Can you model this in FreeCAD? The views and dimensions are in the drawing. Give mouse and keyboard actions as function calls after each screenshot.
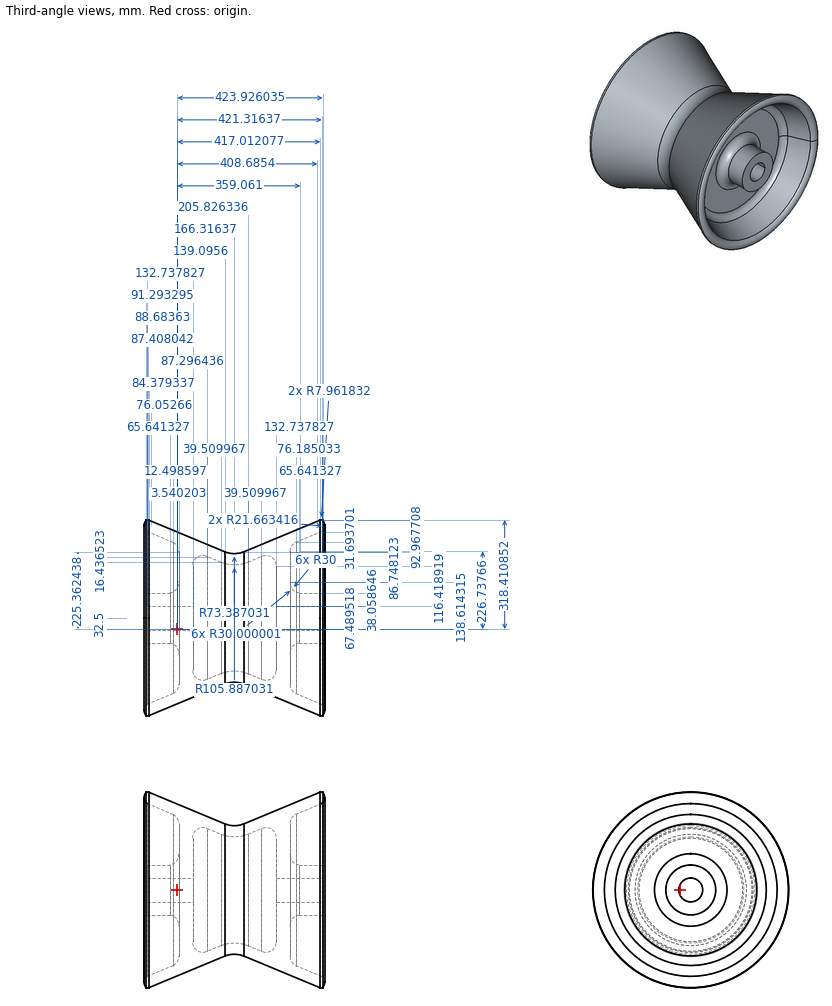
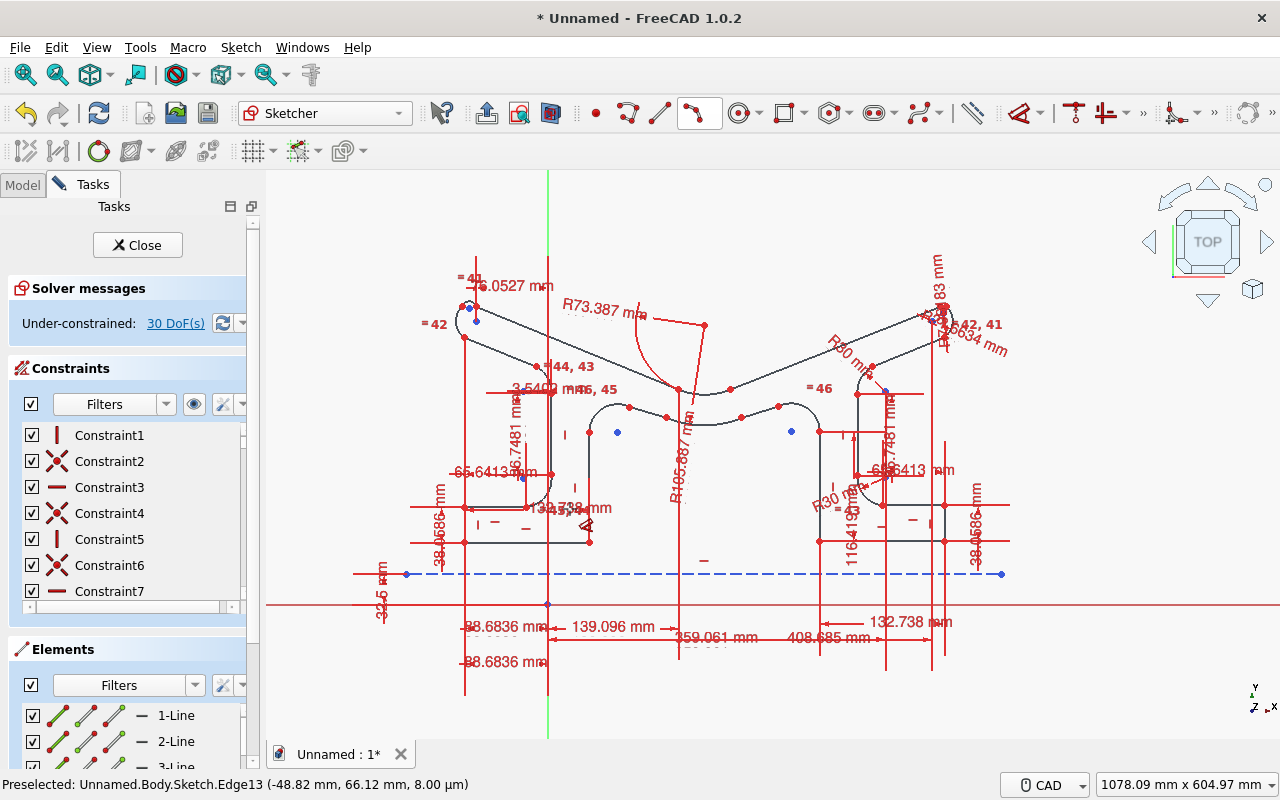
click(589, 510)
click(623, 488)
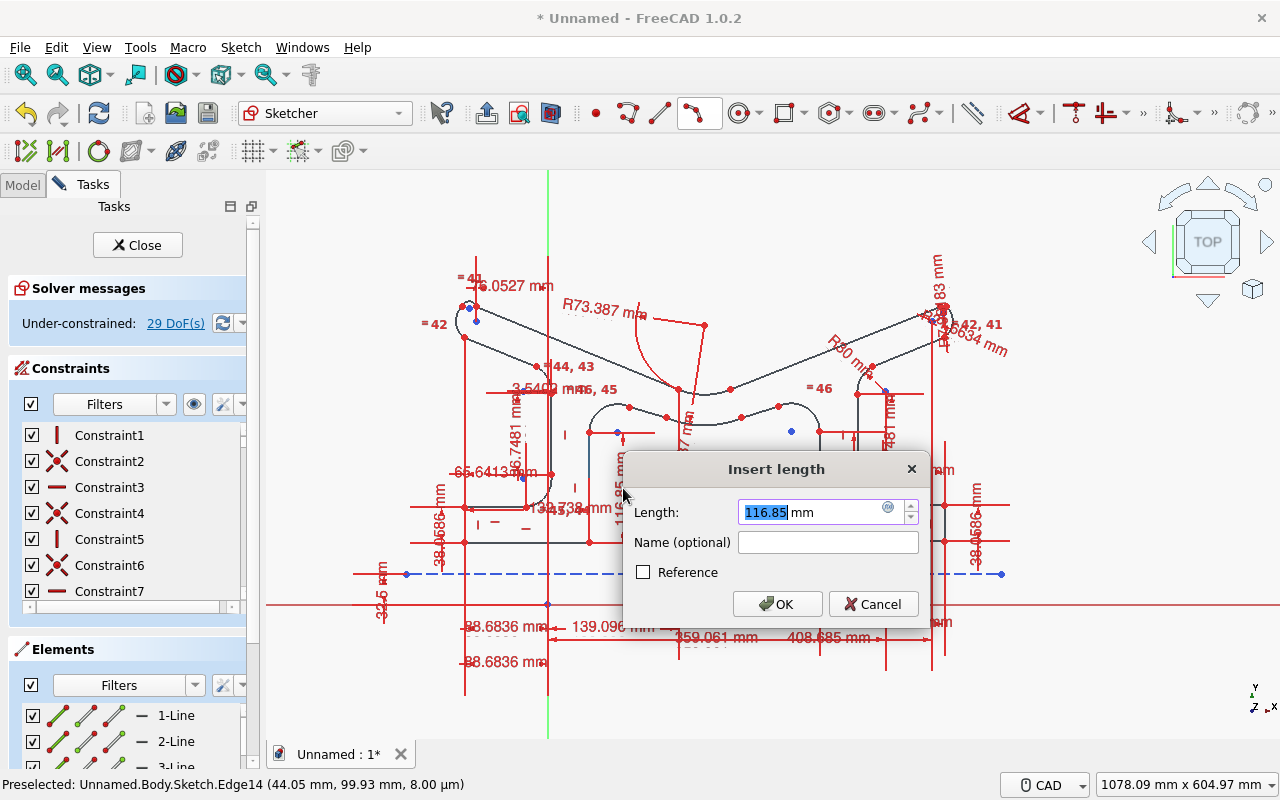
text(116.418919)
key(Return)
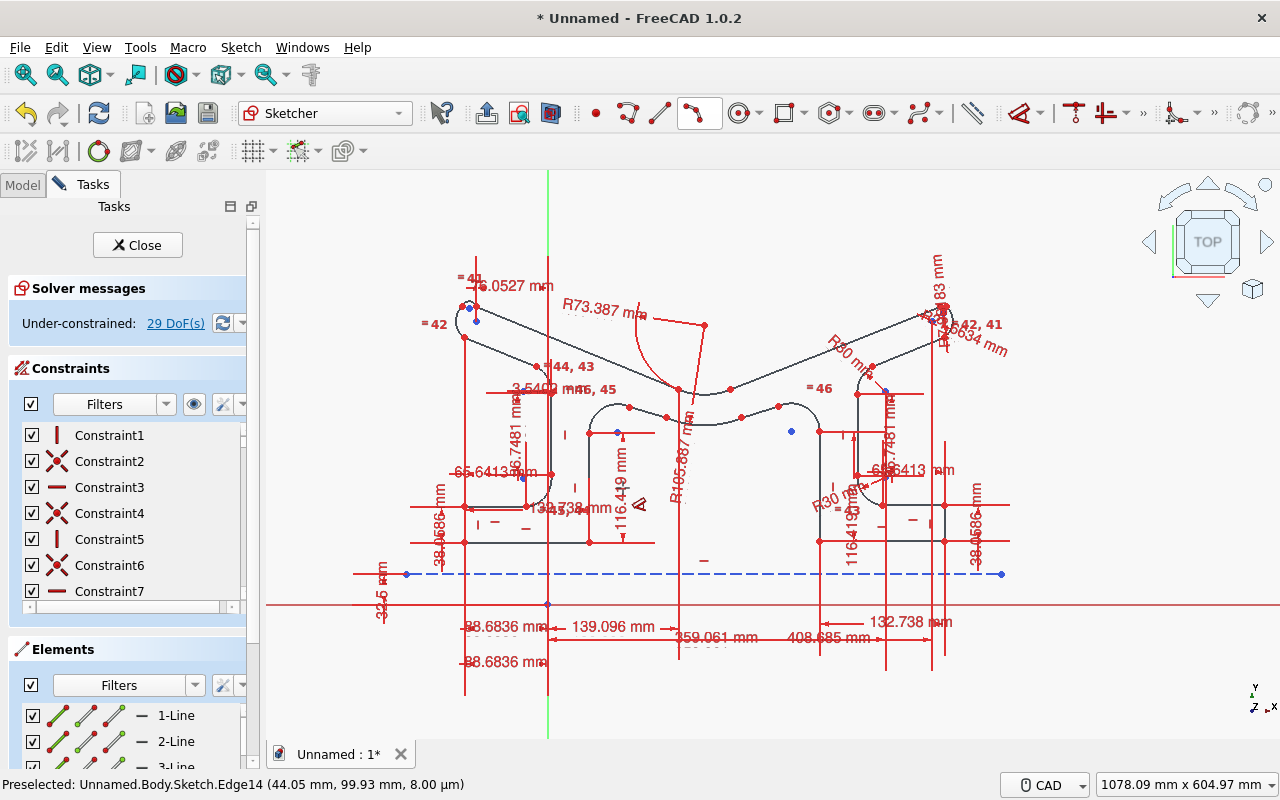
click(820, 541)
click(514, 558)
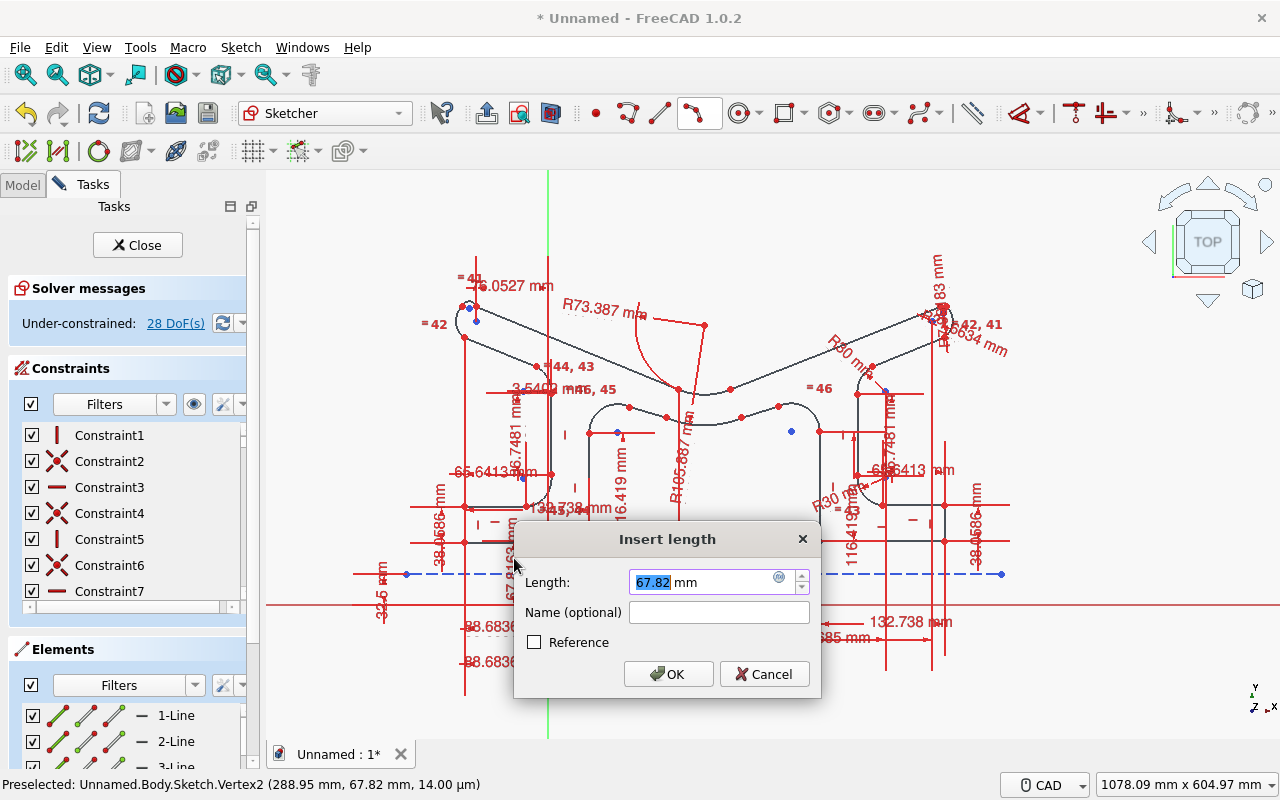
text(67.489518)
key(Return)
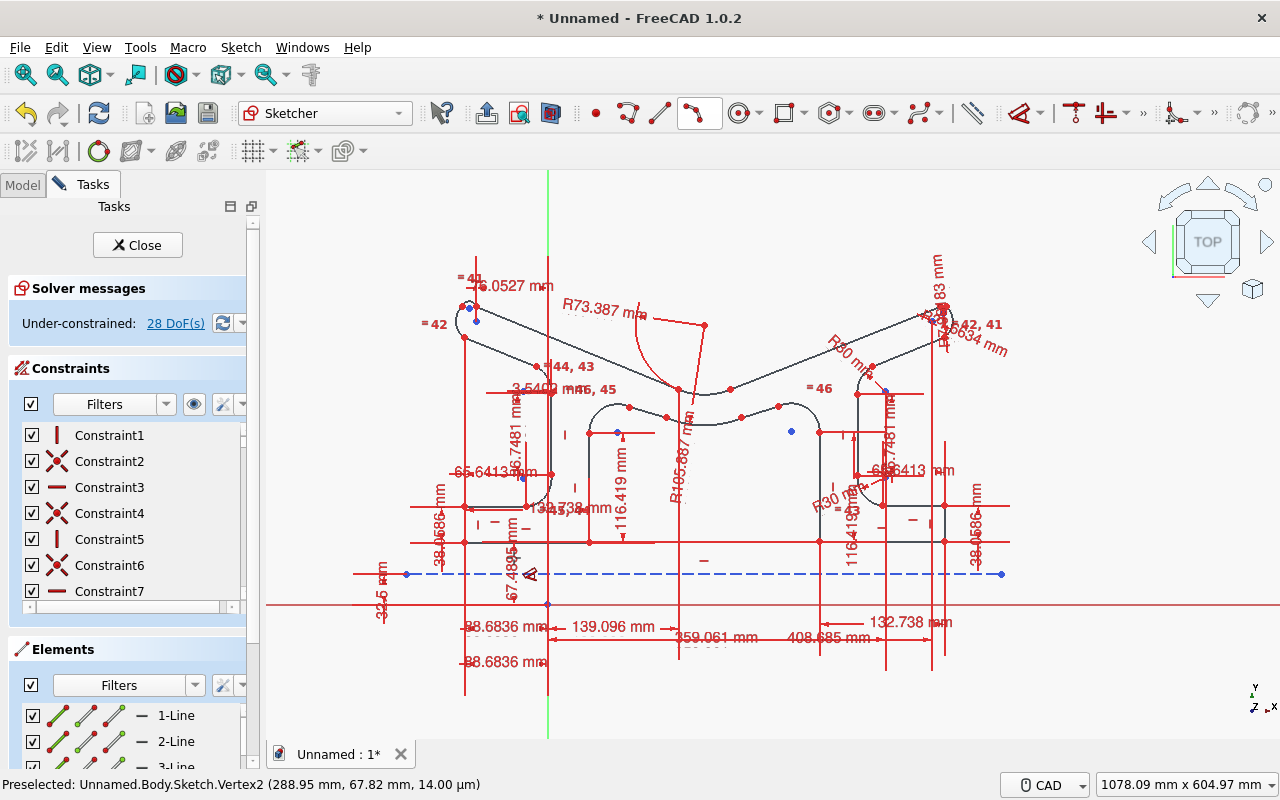
click(945, 542)
click(746, 508)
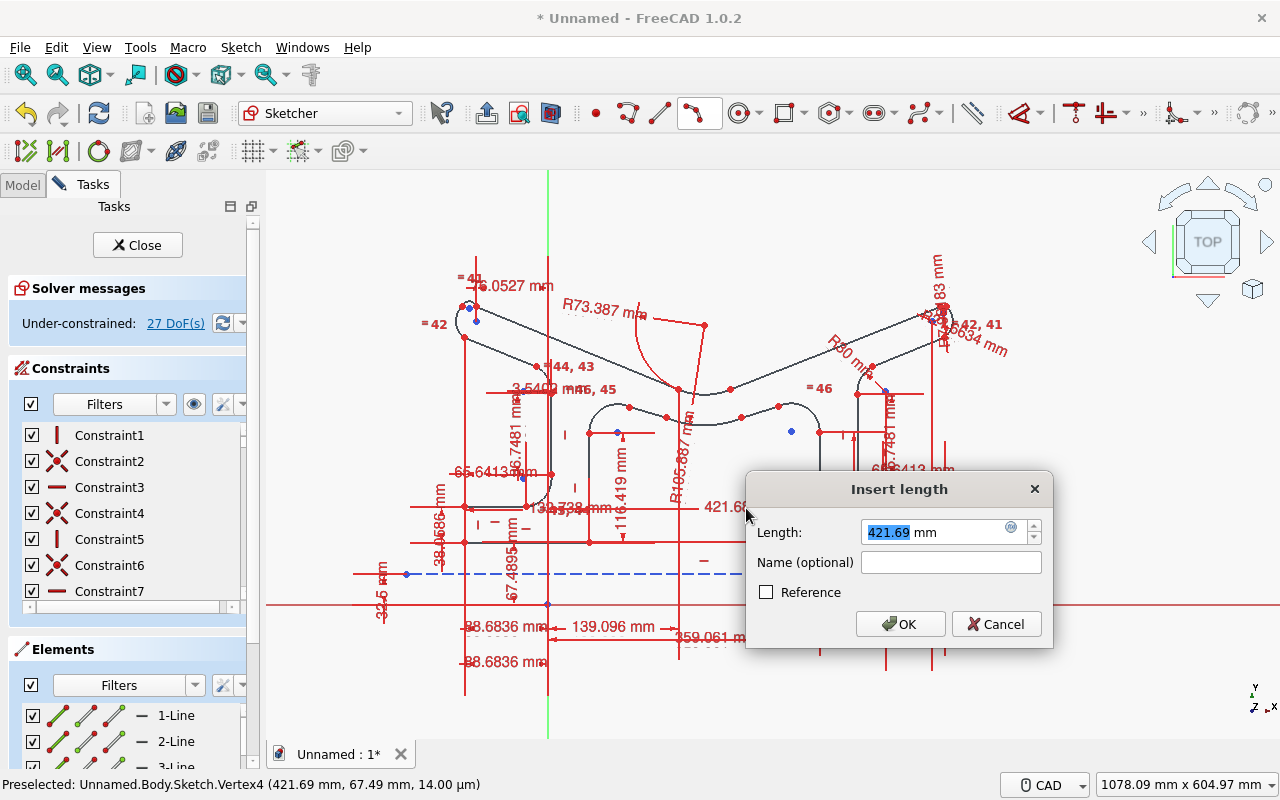
text(421.31637)
key(Return)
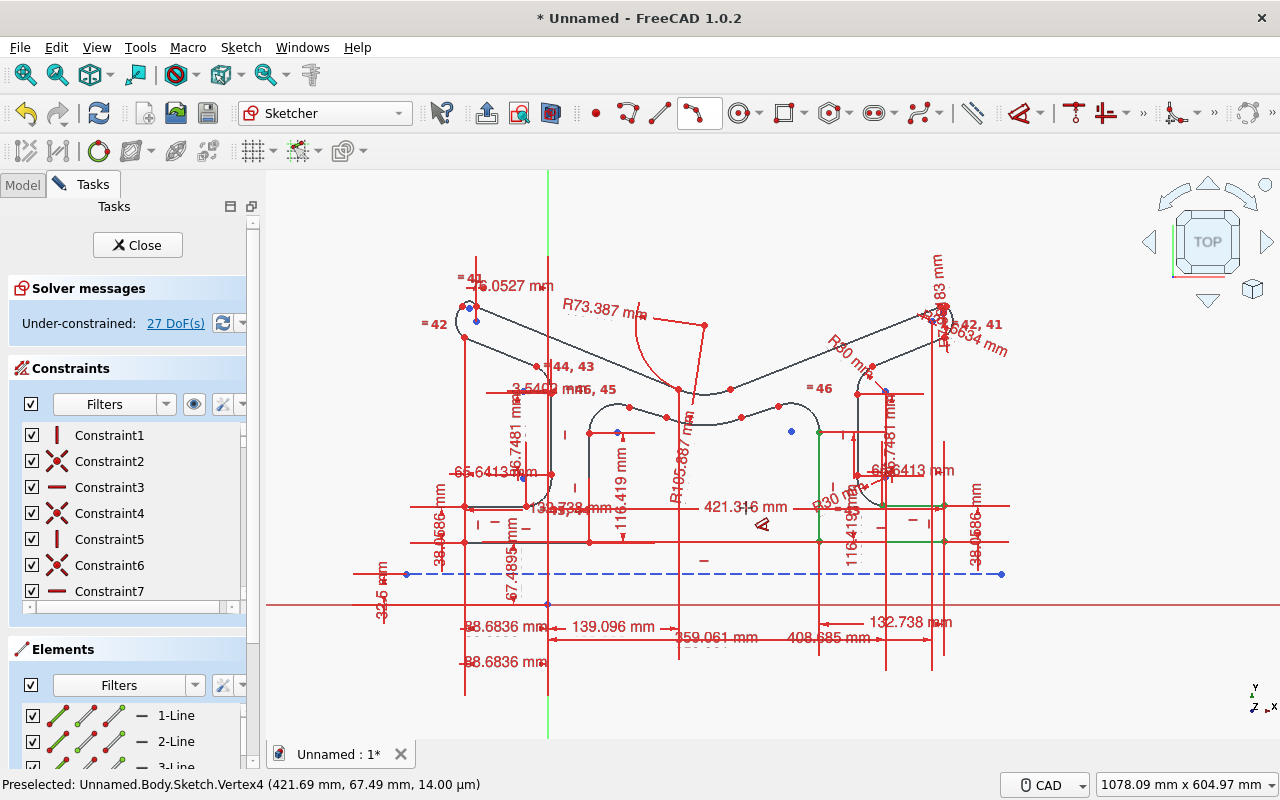
click(944, 338)
click(746, 304)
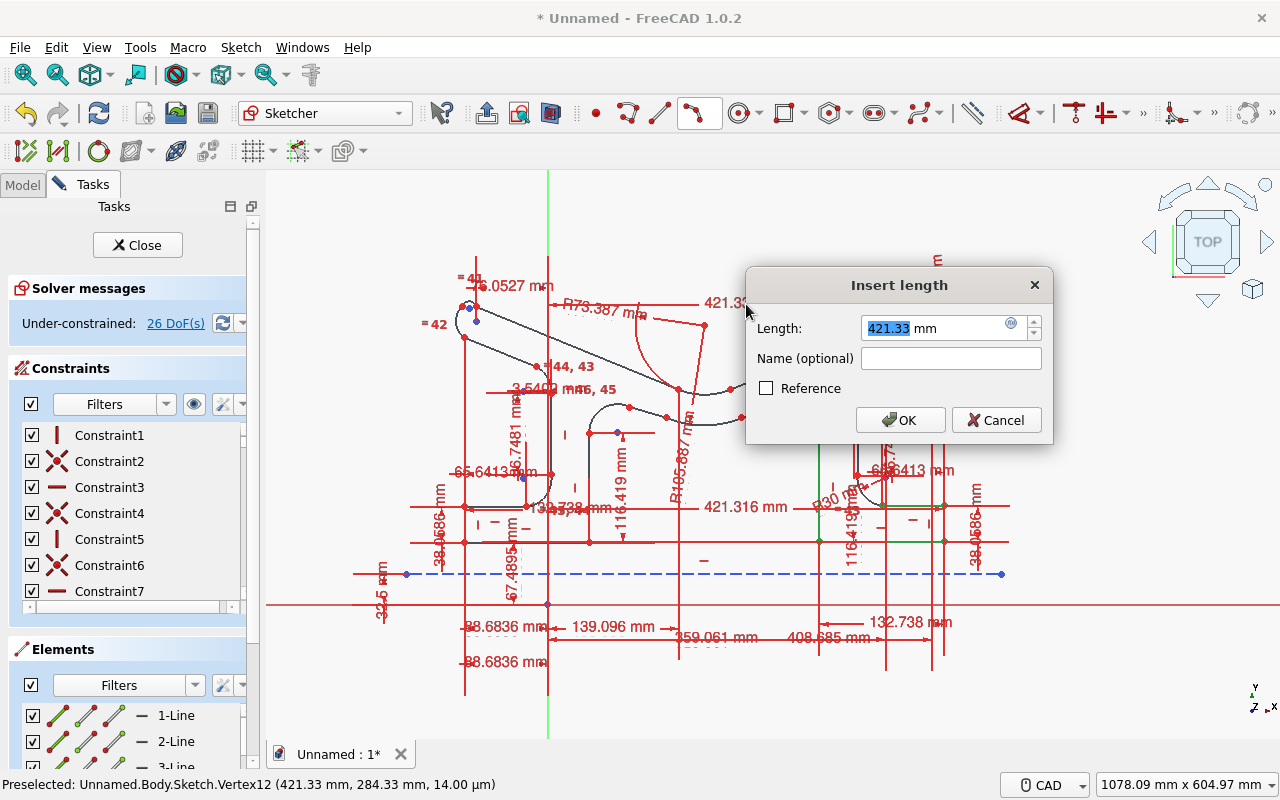
text(421.31637)
key(Return)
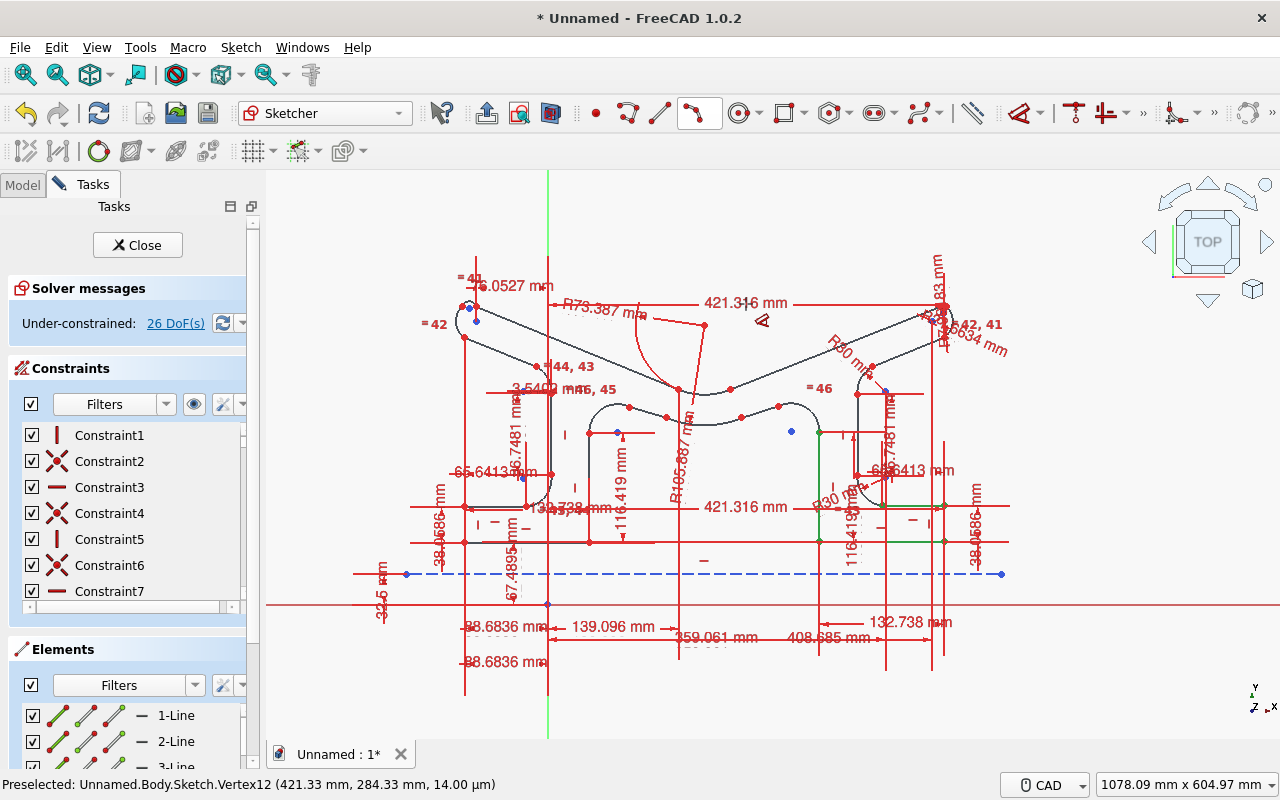
scroll(476, 307, up, 3)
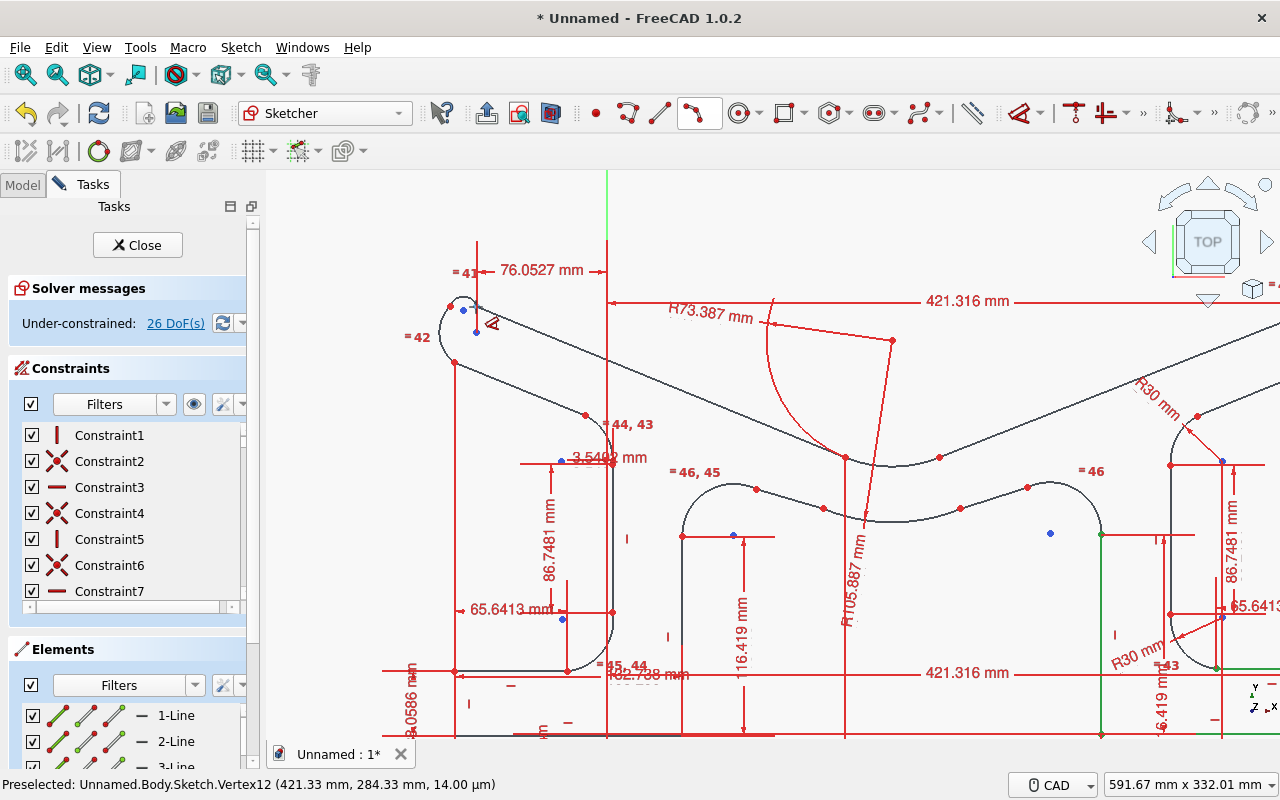
click(477, 307)
click(542, 249)